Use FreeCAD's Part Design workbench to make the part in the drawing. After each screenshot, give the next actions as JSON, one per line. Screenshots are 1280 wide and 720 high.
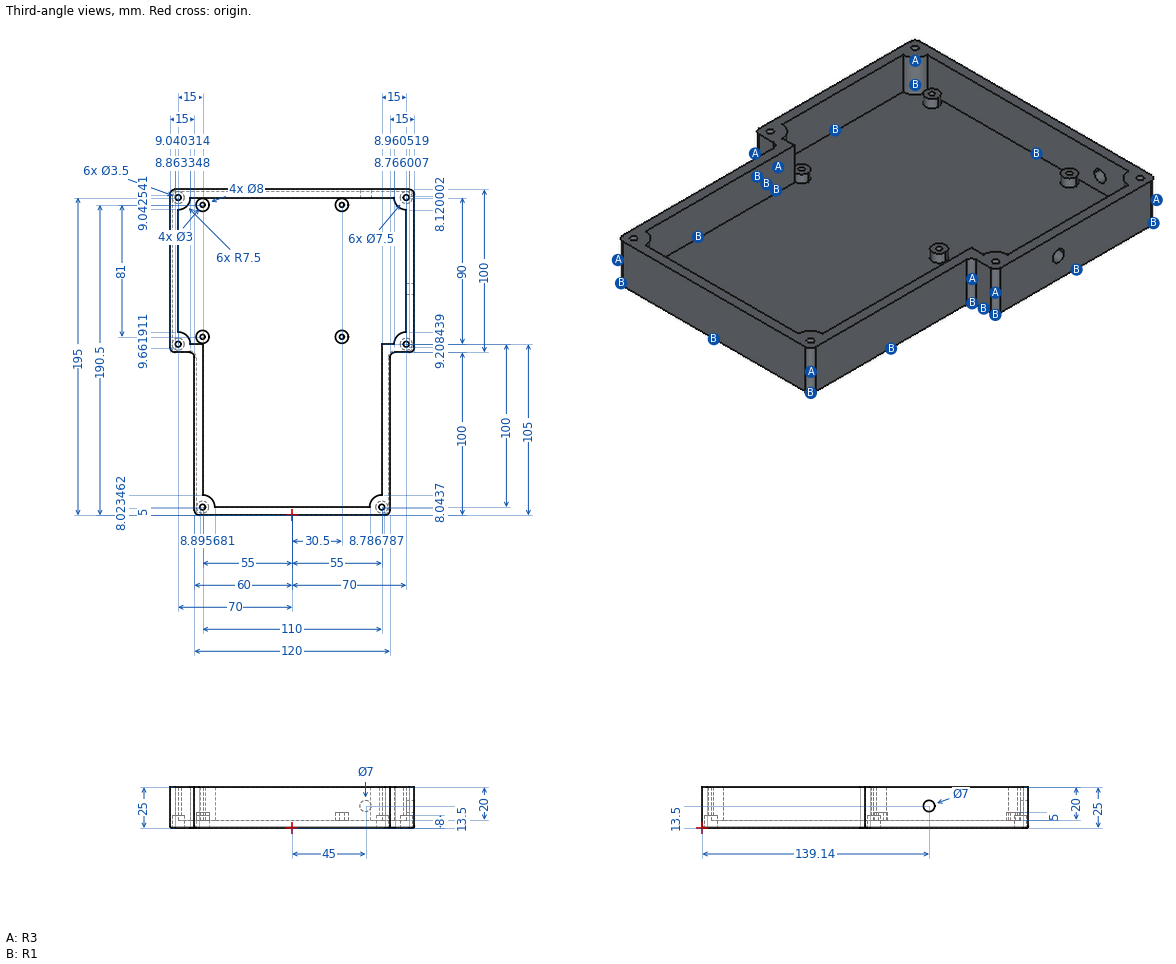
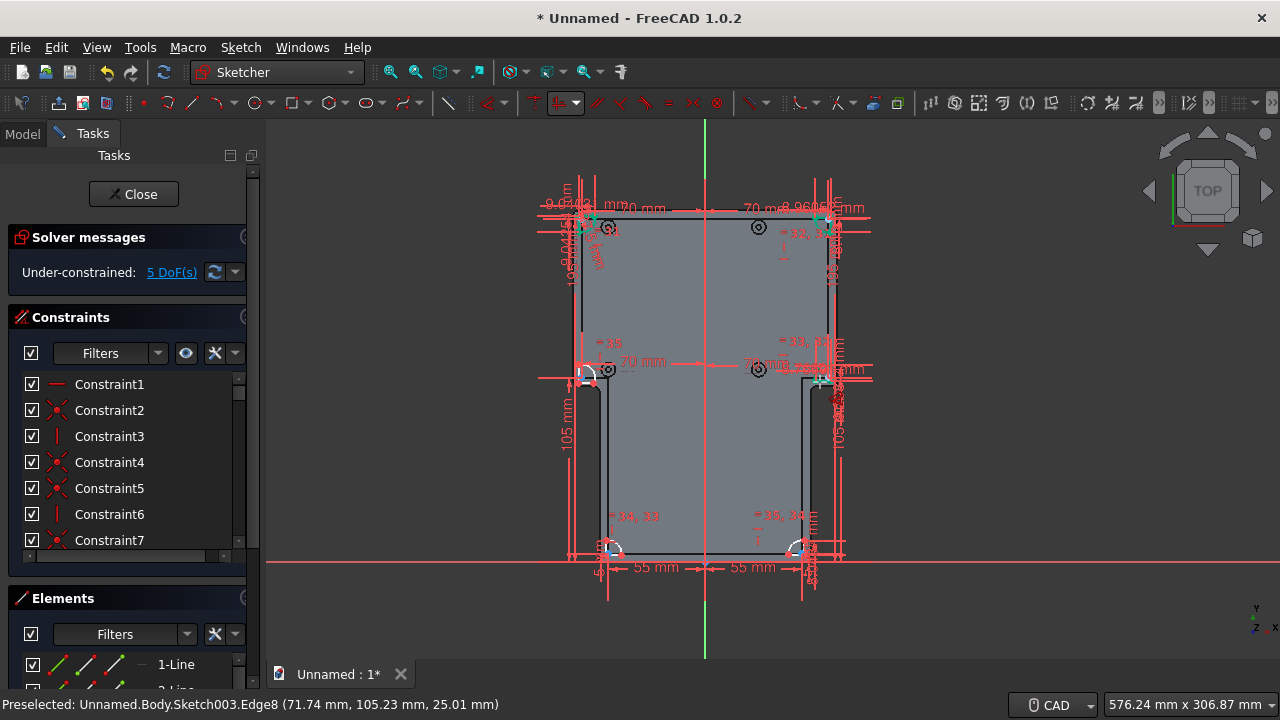
{"action": "scroll", "coordinate": [606, 545], "scroll_direction": "up", "scroll_amount": 6}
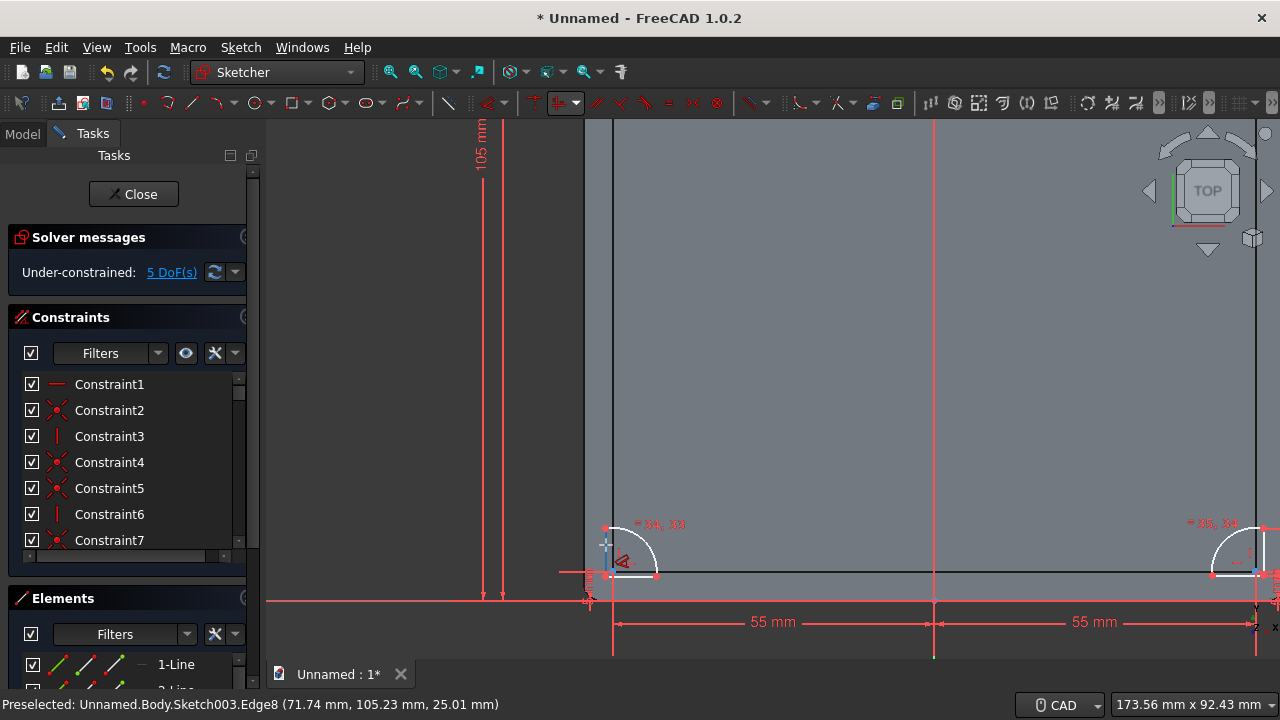
{"action": "left_click", "coordinate": [606, 543]}
{"action": "left_click", "coordinate": [572, 553]}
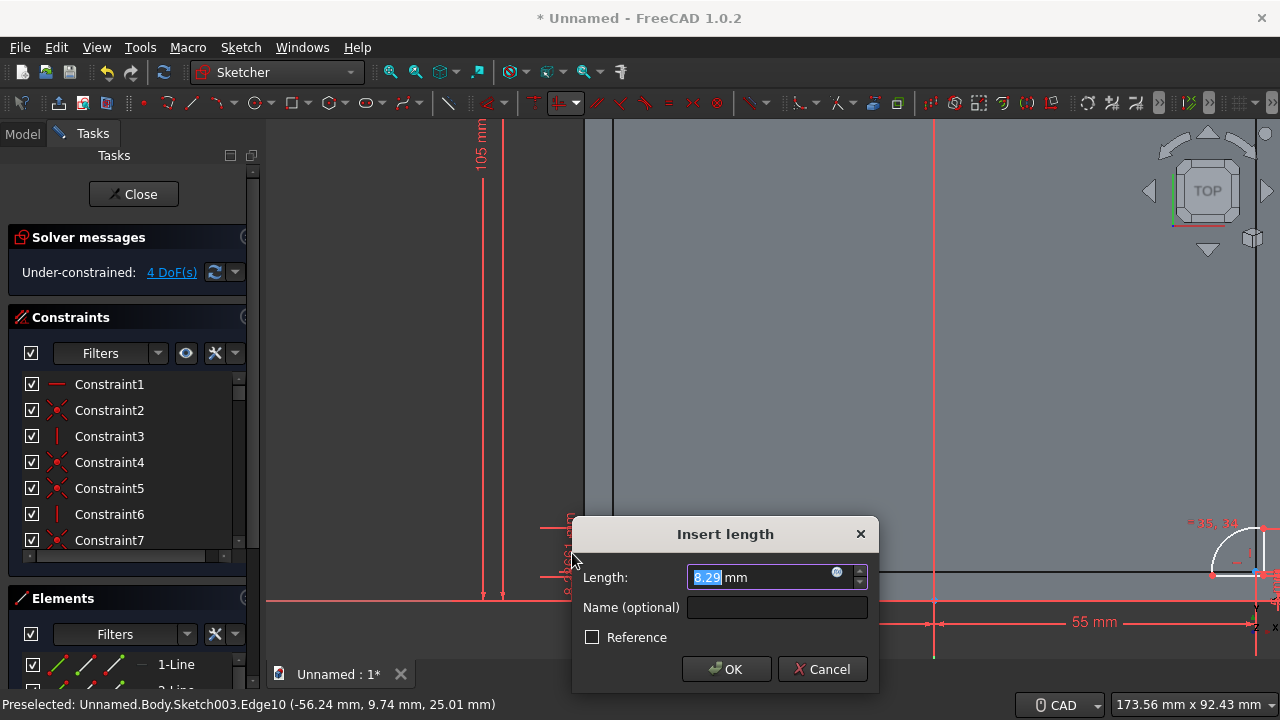
{"action": "type", "text": "8.023462"}
{"action": "key", "text": "Return"}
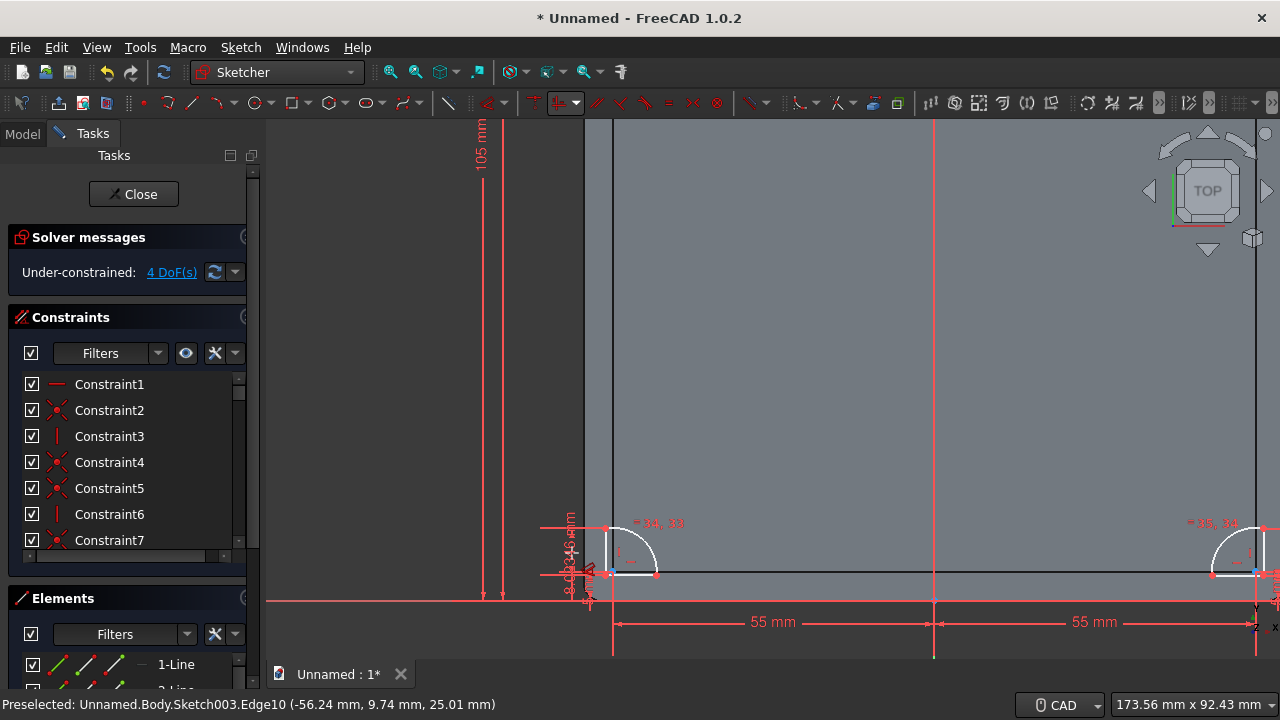
{"action": "left_click", "coordinate": [621, 575]}
{"action": "left_click", "coordinate": [631, 517]}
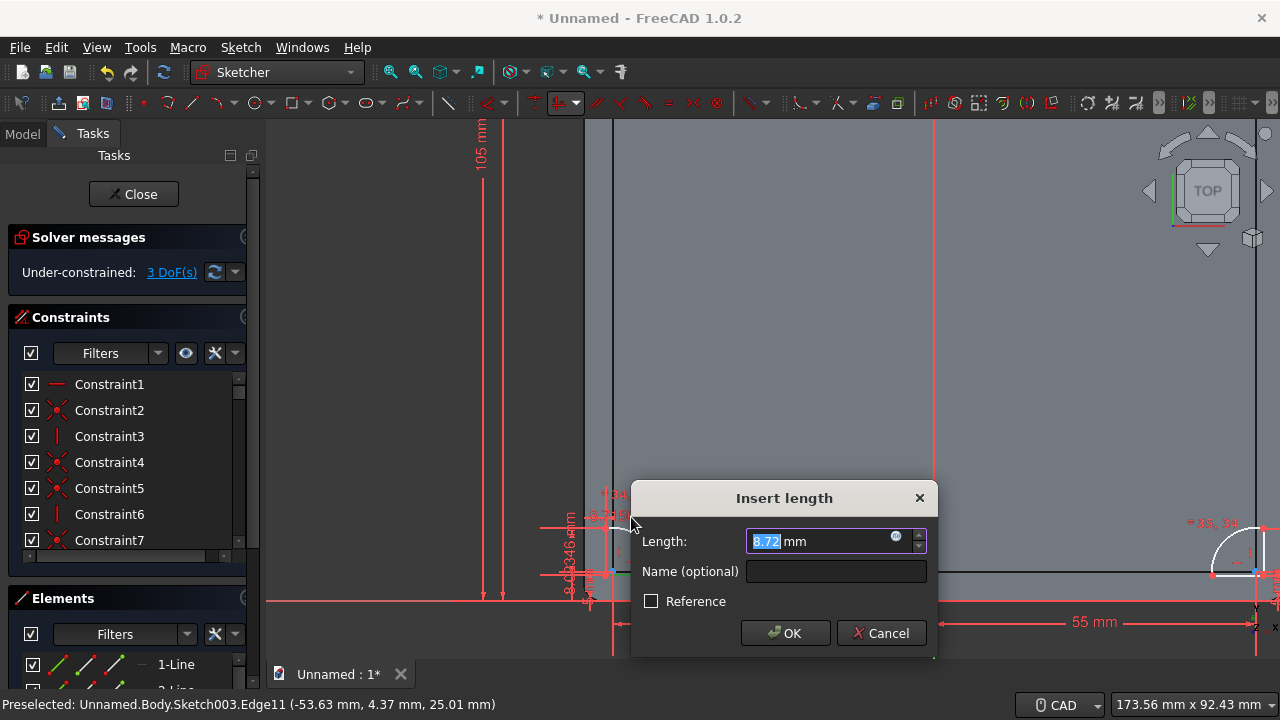
{"action": "type", "text": "8.895681"}
{"action": "key", "text": "Return"}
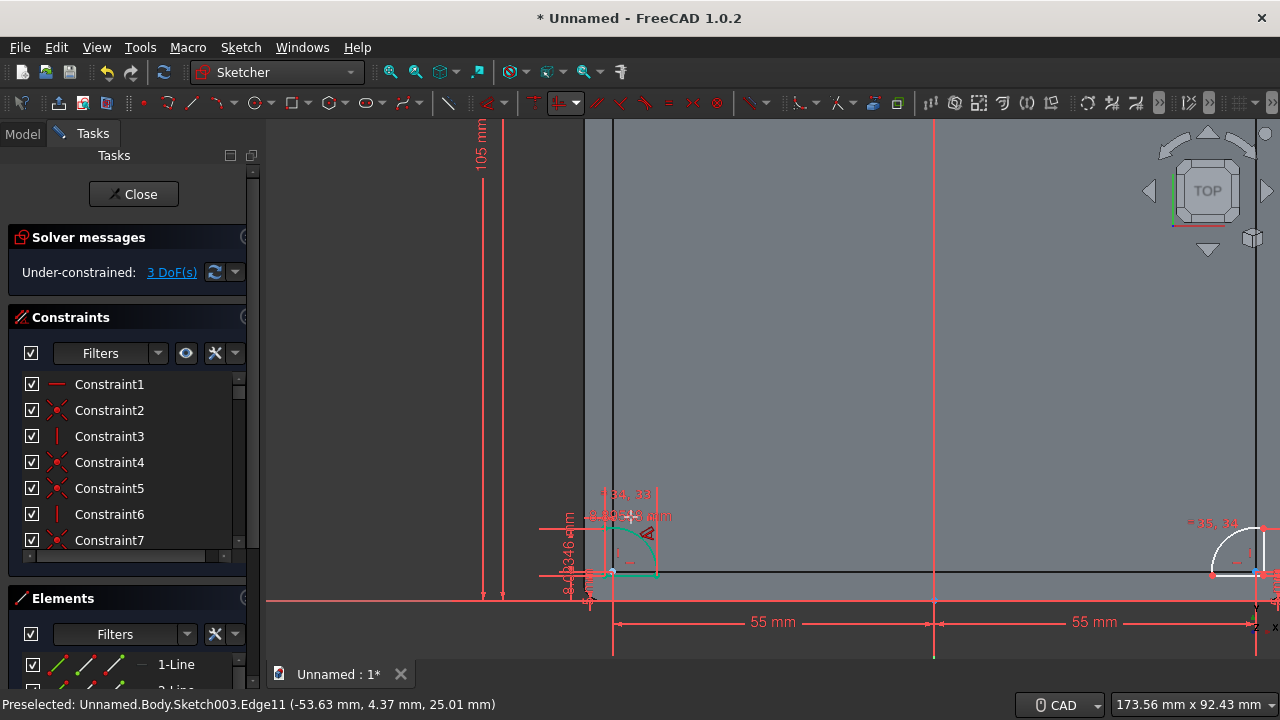
{"action": "scroll", "coordinate": [606, 545], "scroll_direction": "down", "scroll_amount": 6}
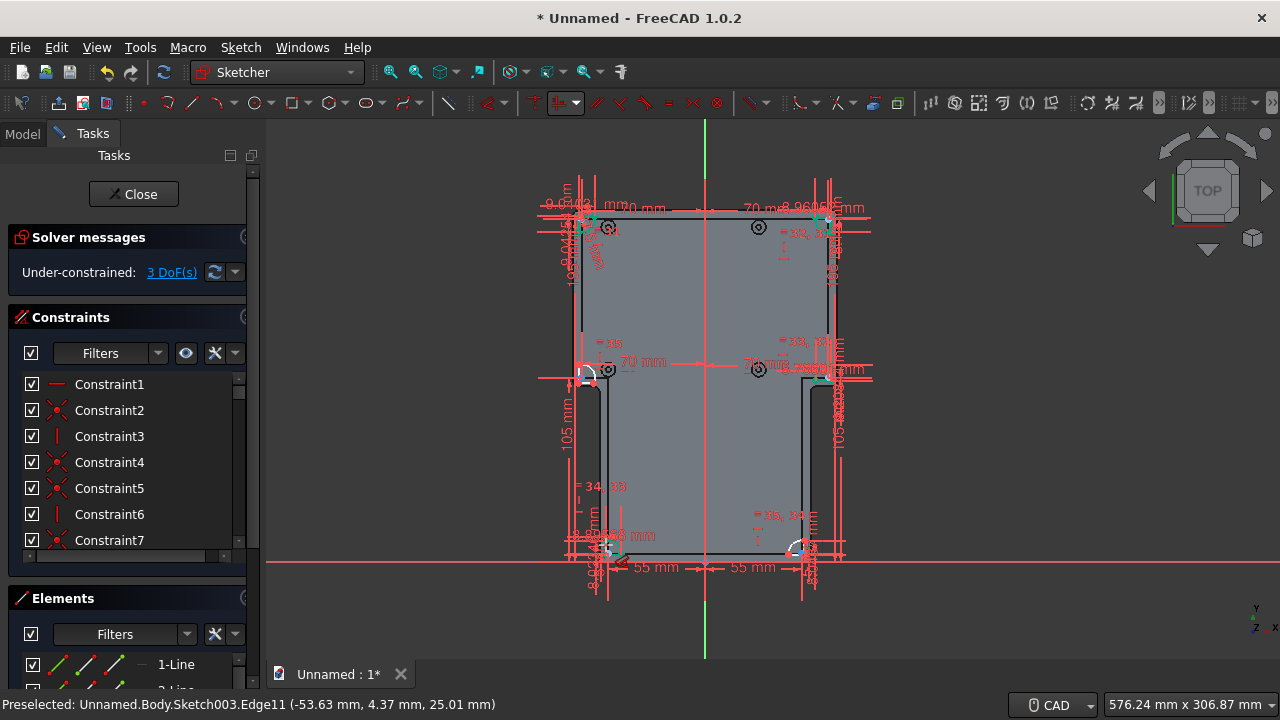
{"action": "scroll", "coordinate": [793, 555], "scroll_direction": "up", "scroll_amount": 6}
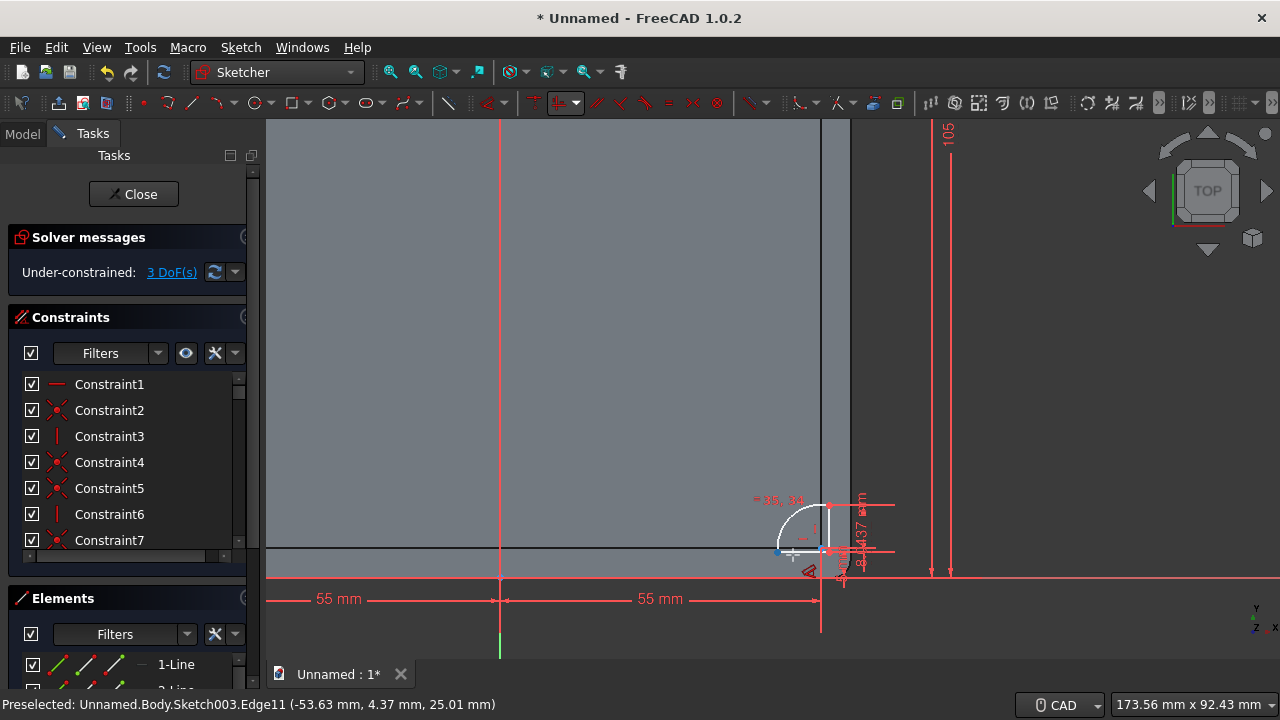
{"action": "left_click", "coordinate": [793, 552]}
{"action": "left_click", "coordinate": [804, 610]}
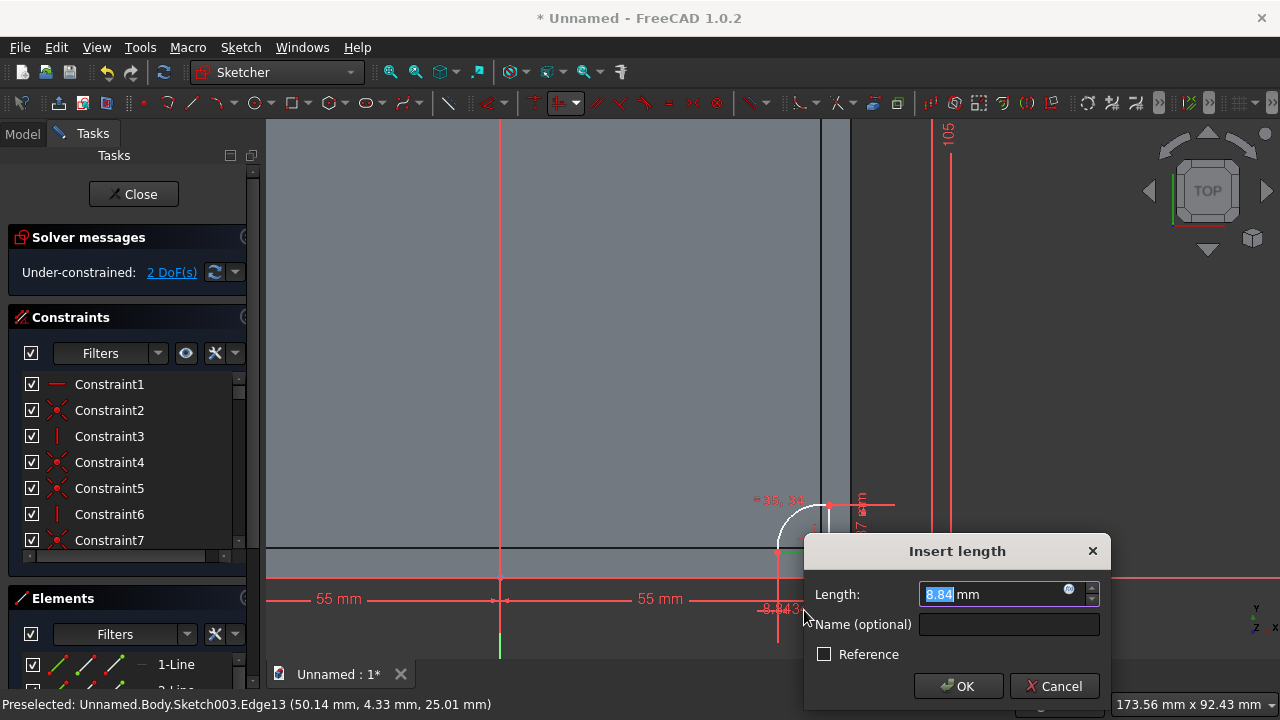
{"action": "type", "text": "8.786787"}
{"action": "key", "text": "Return"}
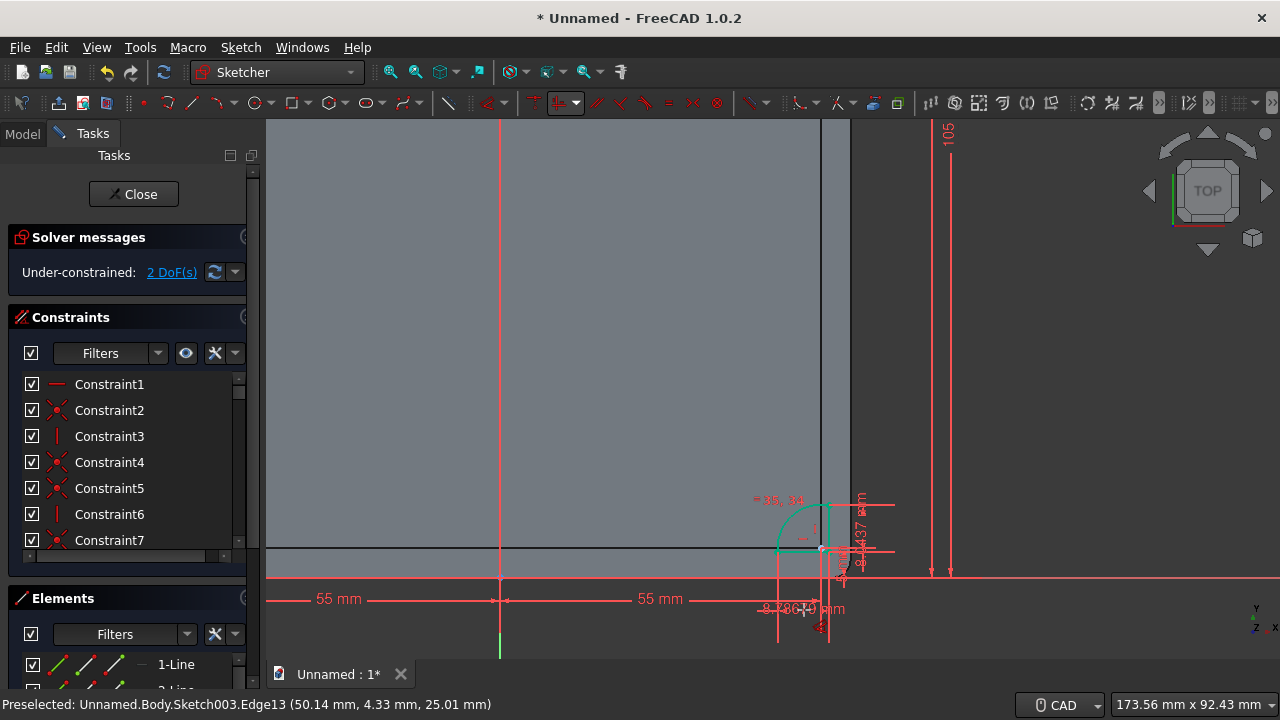
{"action": "scroll", "coordinate": [793, 555], "scroll_direction": "down", "scroll_amount": 6}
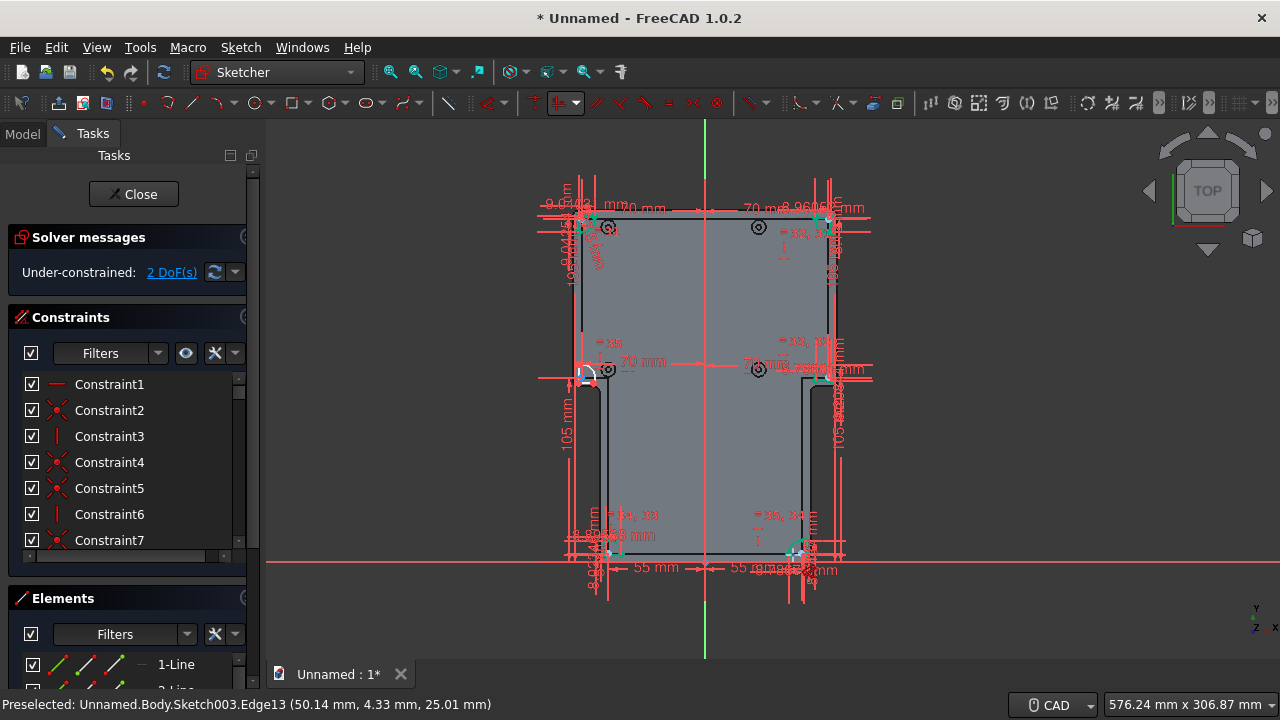
{"action": "scroll", "coordinate": [579, 370], "scroll_direction": "up", "scroll_amount": 5}